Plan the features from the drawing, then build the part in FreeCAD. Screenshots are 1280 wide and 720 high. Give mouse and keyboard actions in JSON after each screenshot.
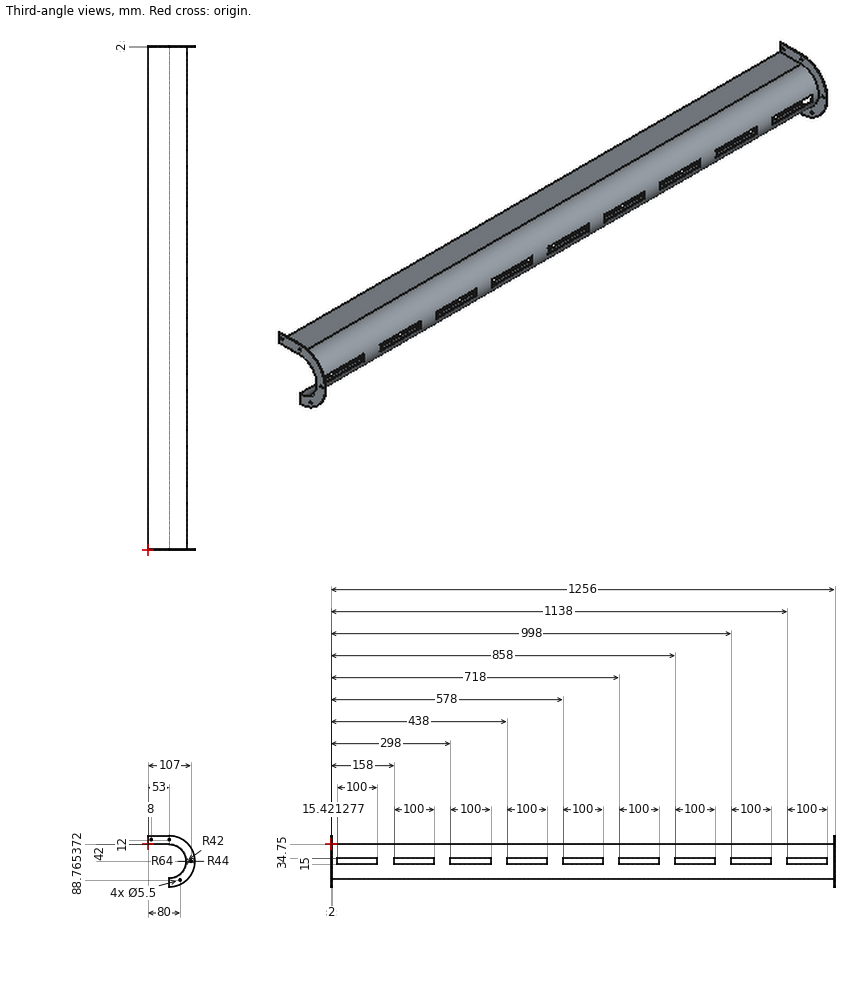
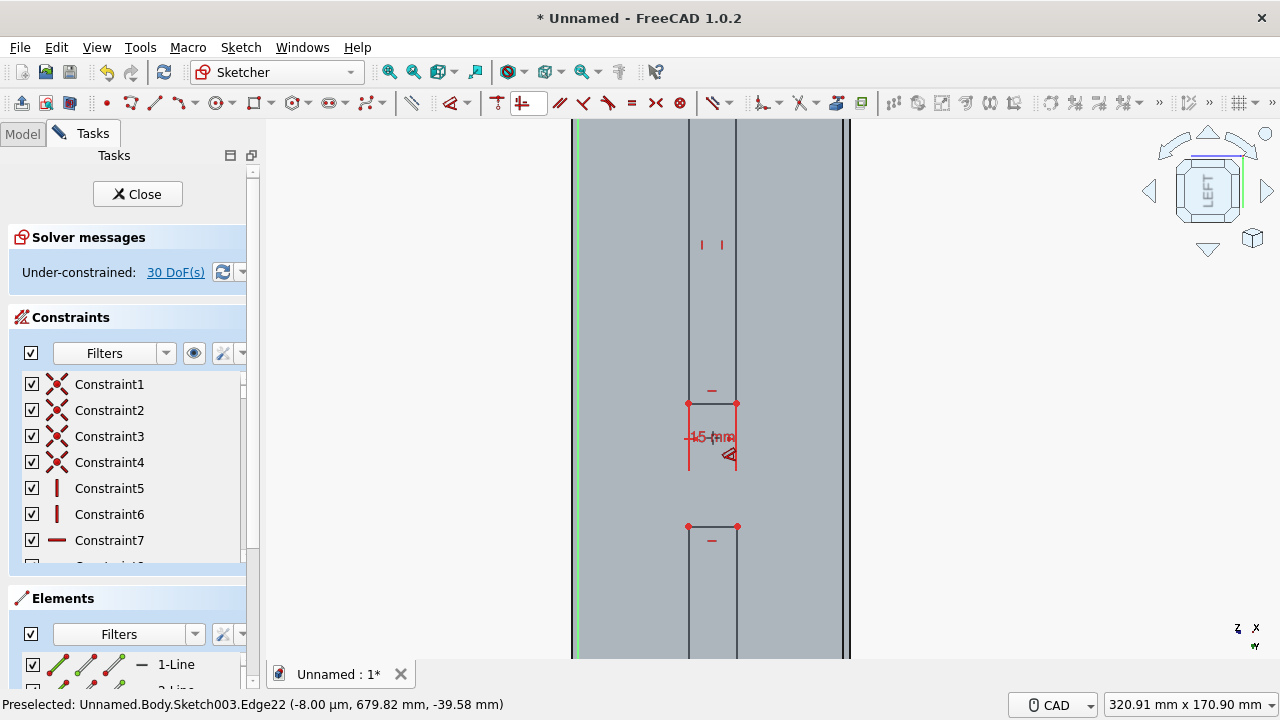
{"action": "scroll", "coordinate": [709, 407], "scroll_direction": "down", "scroll_amount": 12}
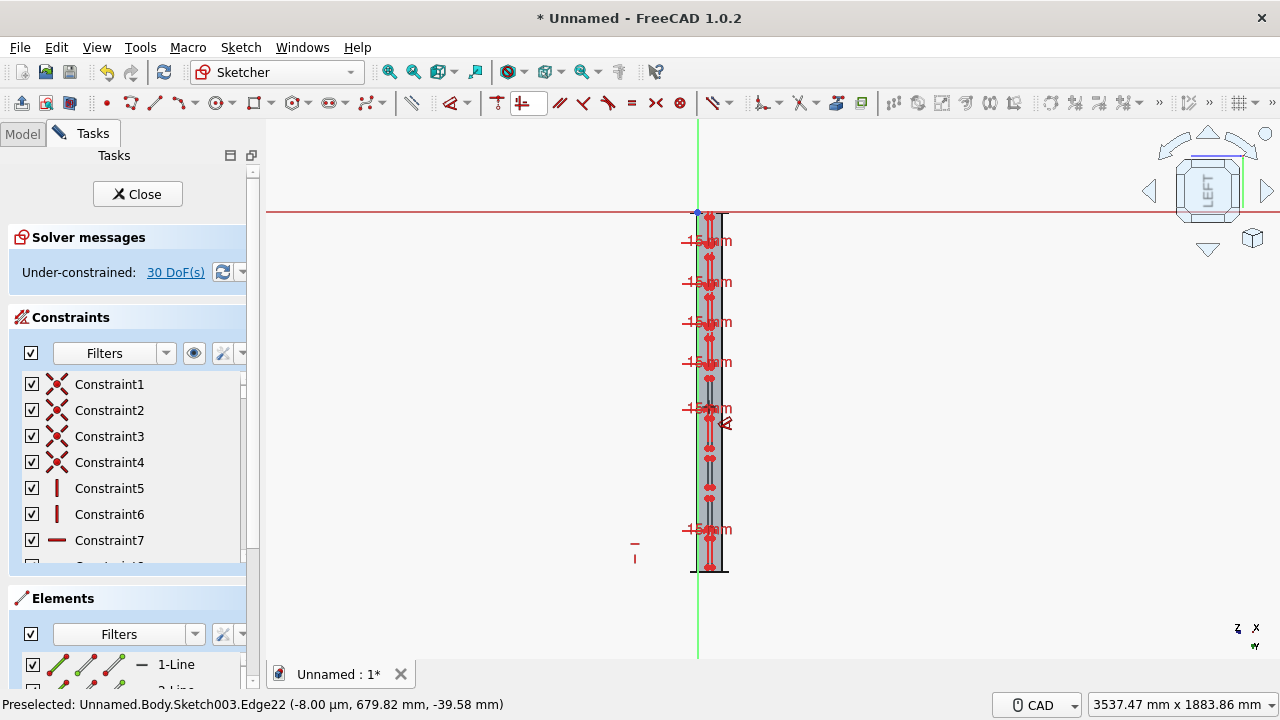
{"action": "scroll", "coordinate": [709, 448], "scroll_direction": "up", "scroll_amount": 12}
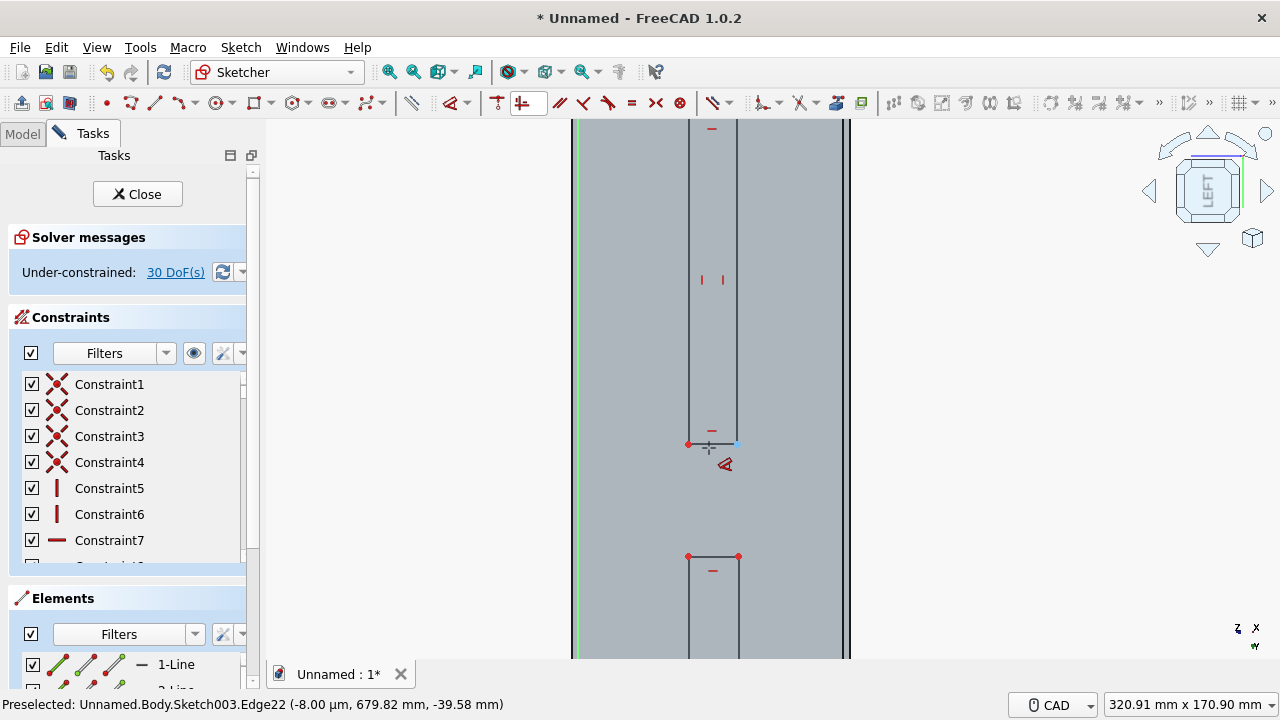
{"action": "left_click", "coordinate": [703, 444]}
{"action": "left_click", "coordinate": [713, 478]}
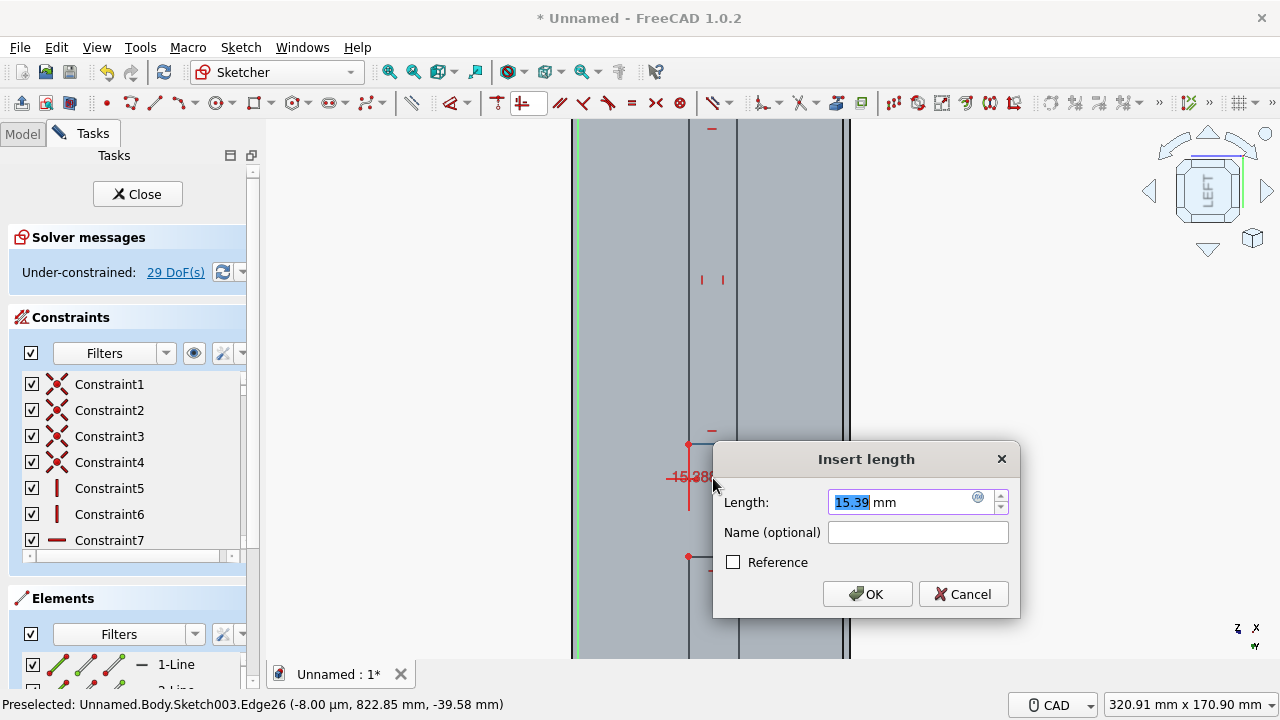
{"action": "type", "text": "15"}
{"action": "key", "text": "Return"}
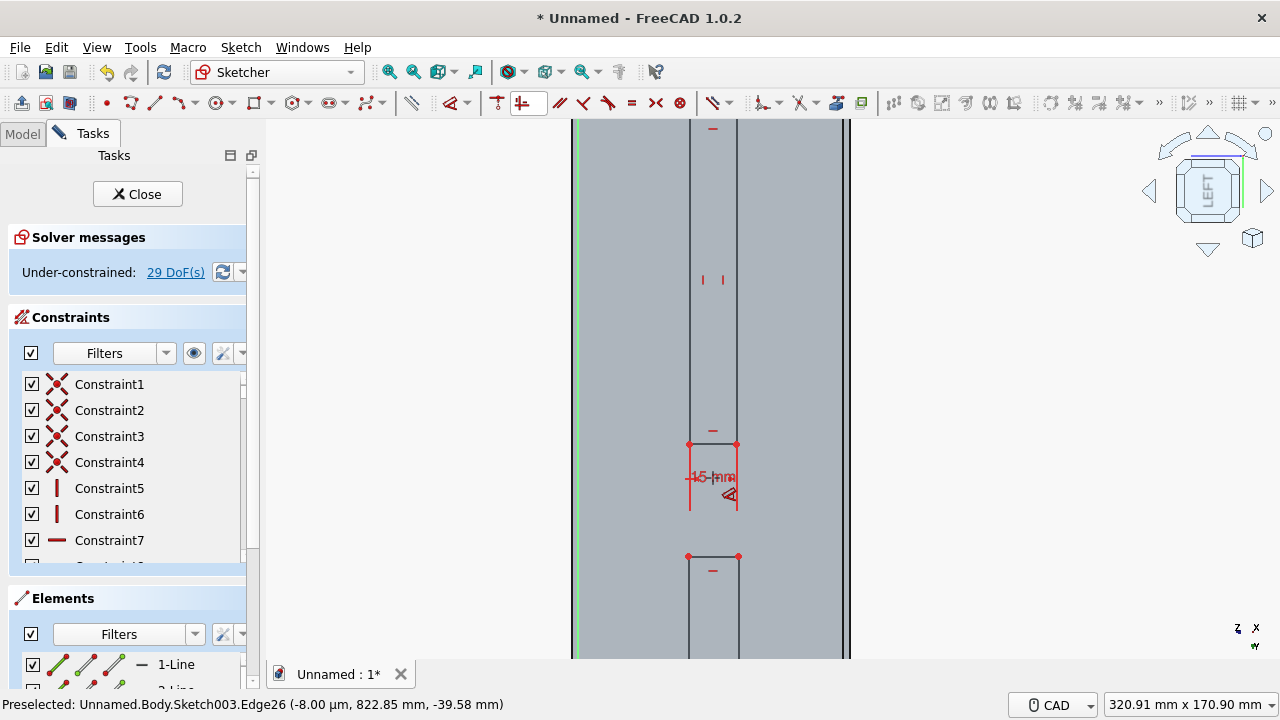
{"action": "scroll", "coordinate": [709, 448], "scroll_direction": "down", "scroll_amount": 12}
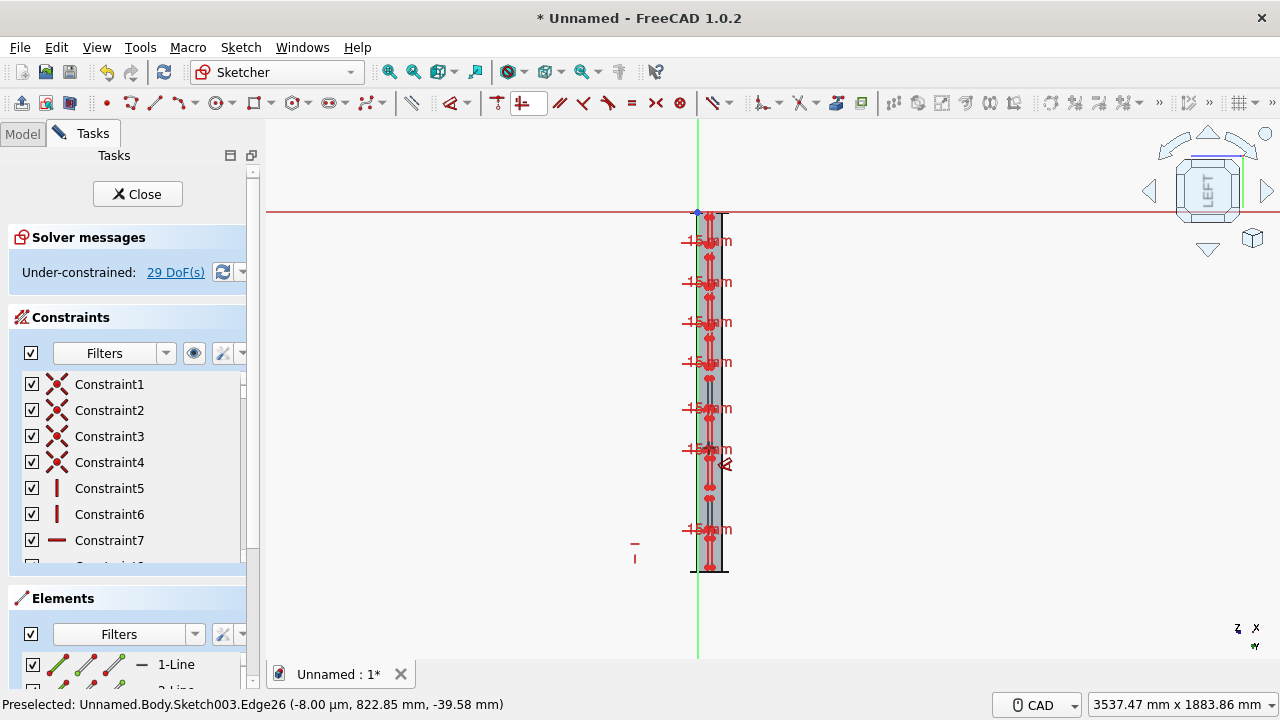
{"action": "scroll", "coordinate": [709, 487], "scroll_direction": "up", "scroll_amount": 12}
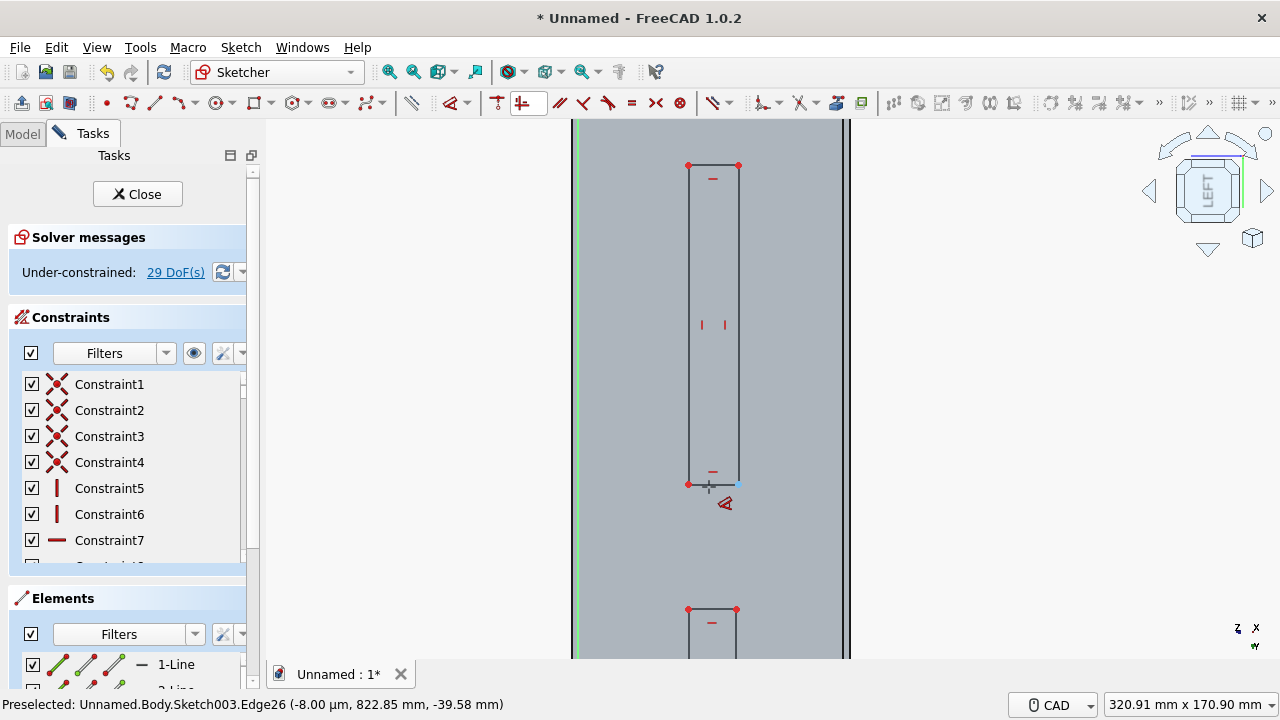
{"action": "left_click", "coordinate": [704, 485]}
{"action": "left_click", "coordinate": [714, 519]}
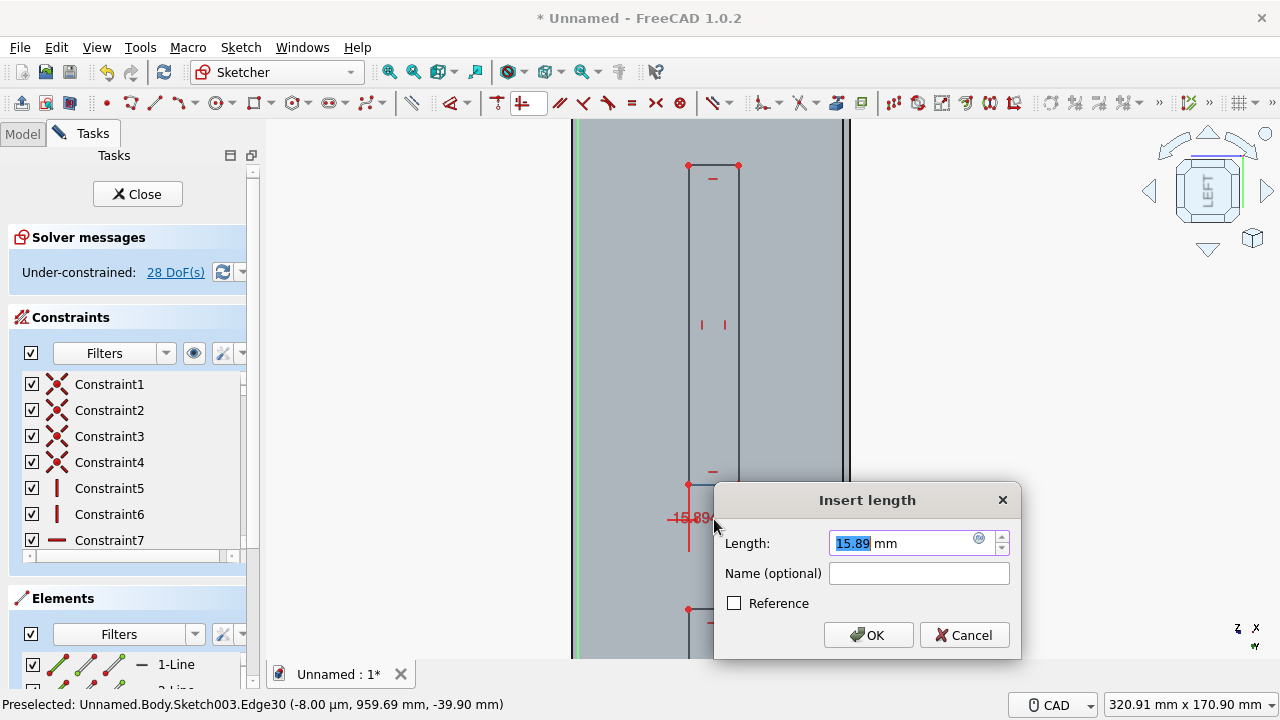
{"action": "type", "text": "15"}
{"action": "key", "text": "Return"}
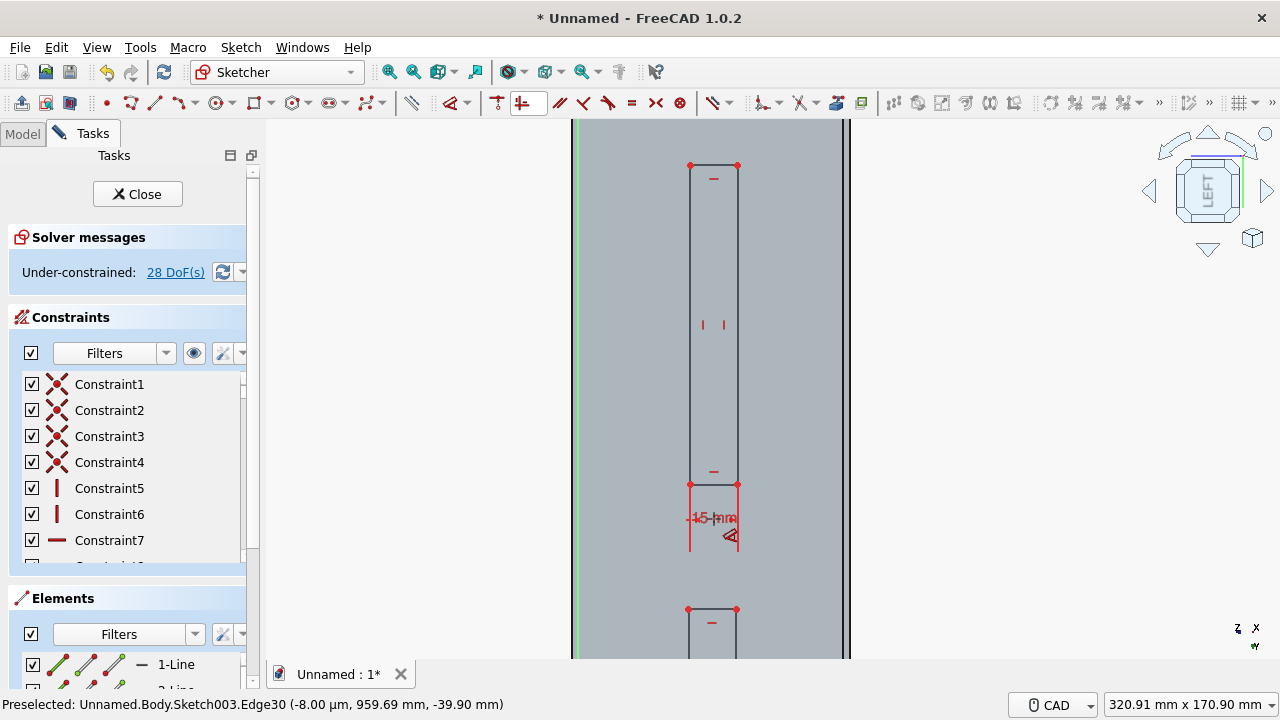
{"action": "scroll", "coordinate": [709, 487], "scroll_direction": "down", "scroll_amount": 12}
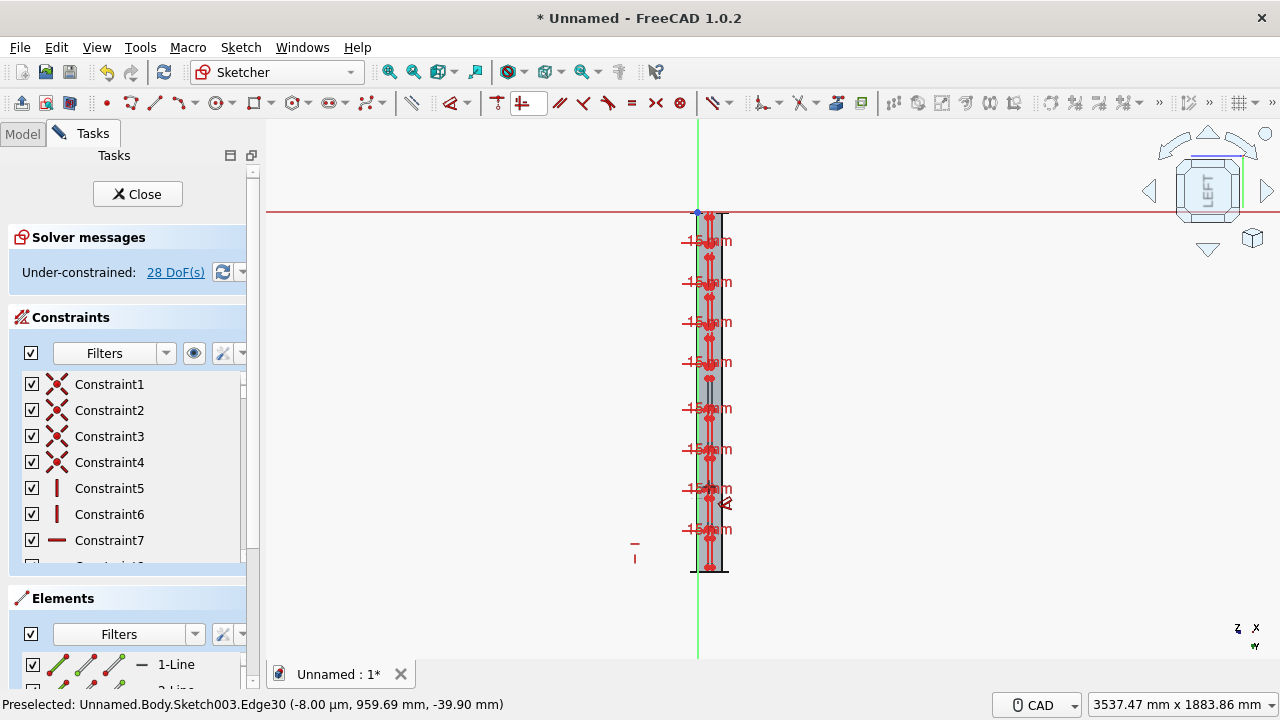
{"action": "scroll", "coordinate": [709, 568], "scroll_direction": "up", "scroll_amount": 12}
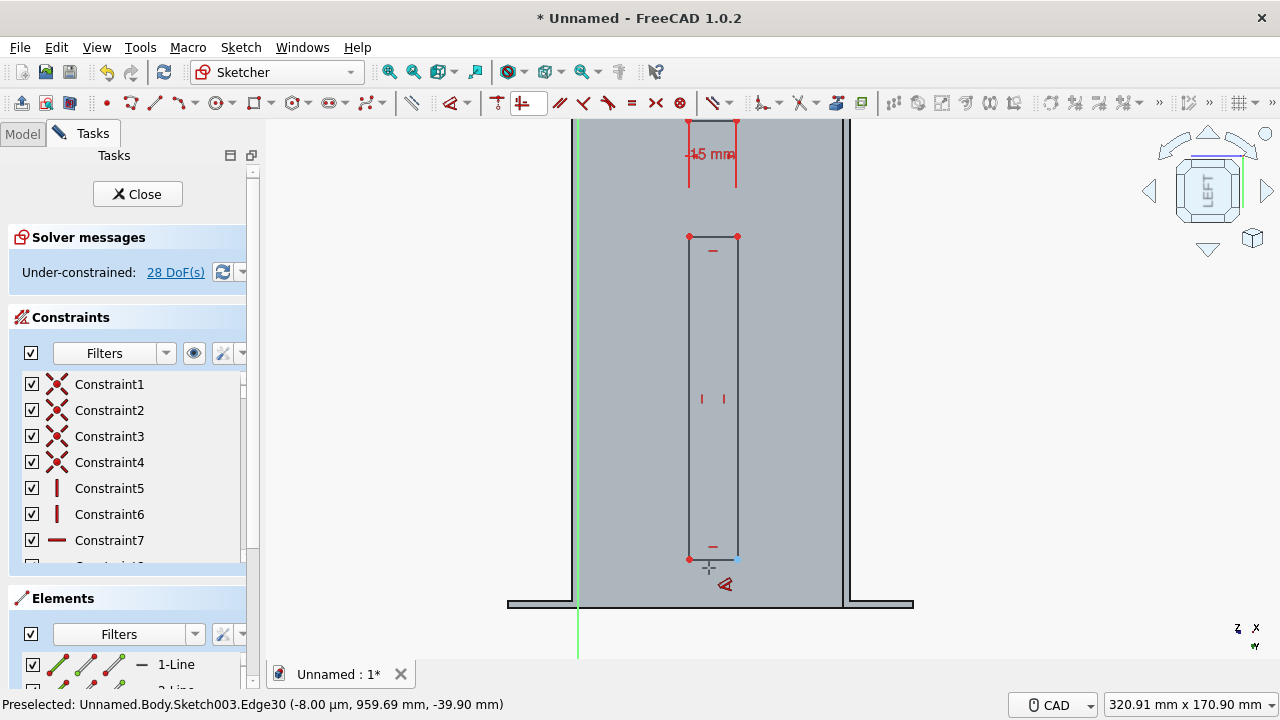
{"action": "left_click", "coordinate": [704, 560]}
{"action": "left_click", "coordinate": [713, 594]}